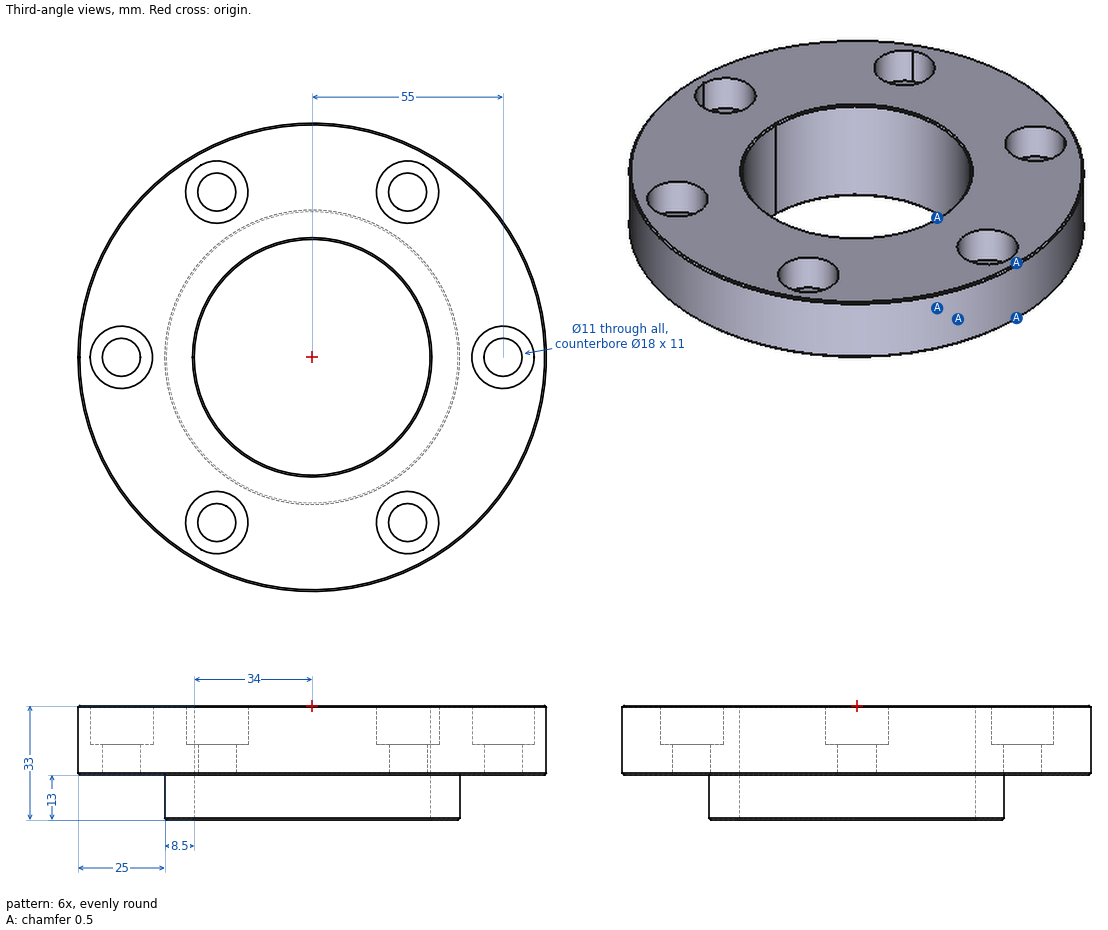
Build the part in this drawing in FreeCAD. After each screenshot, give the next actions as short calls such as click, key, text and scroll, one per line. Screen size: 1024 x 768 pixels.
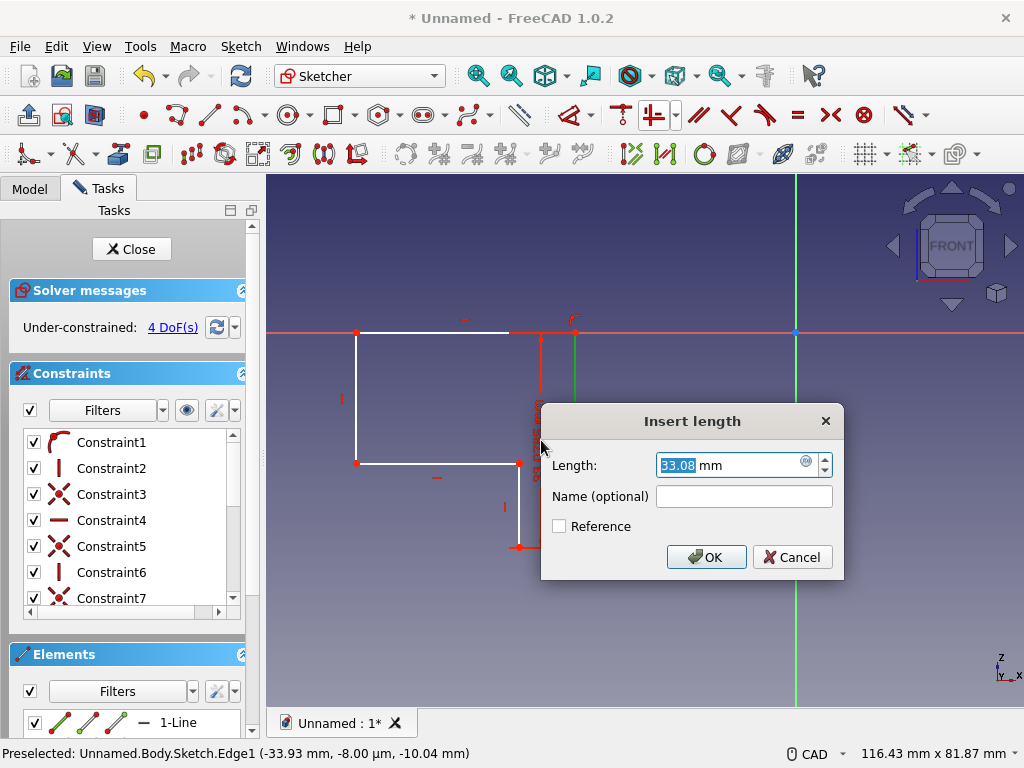
text(33)
key(Return)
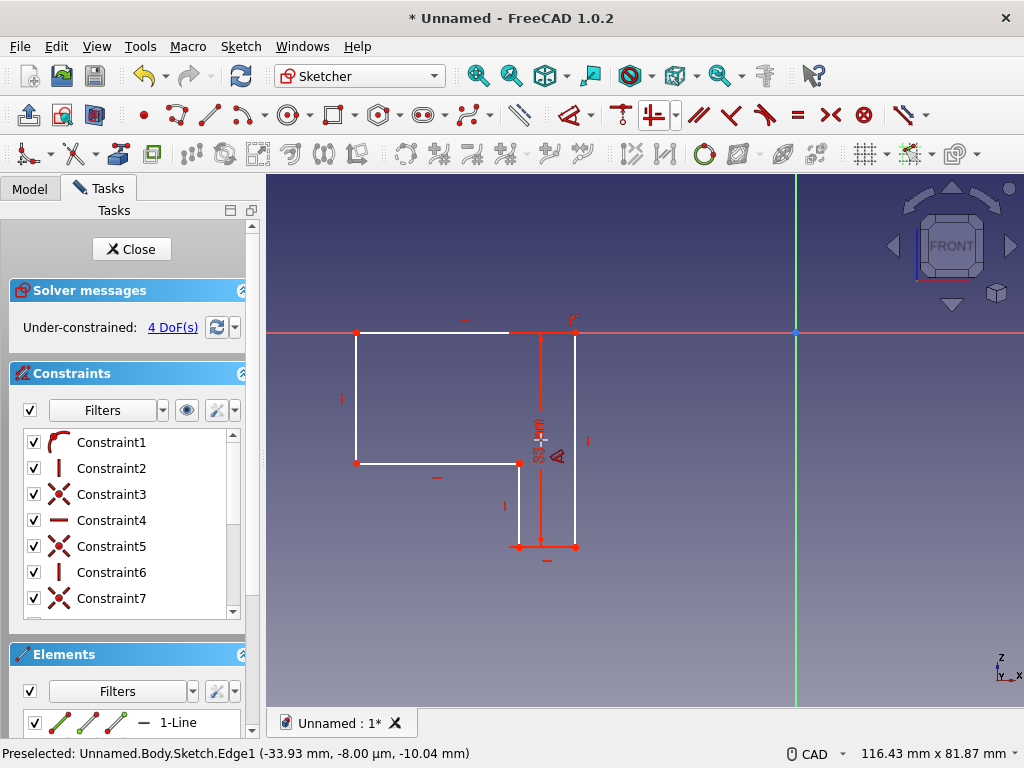
click(519, 522)
click(485, 506)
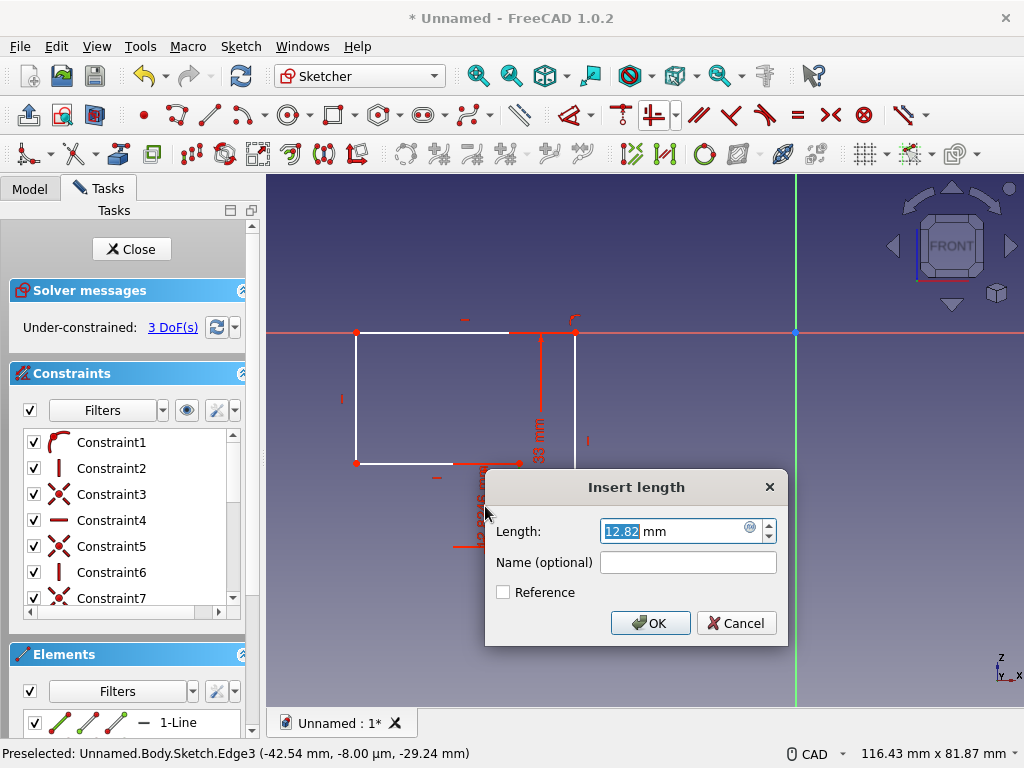
text(13)
key(Return)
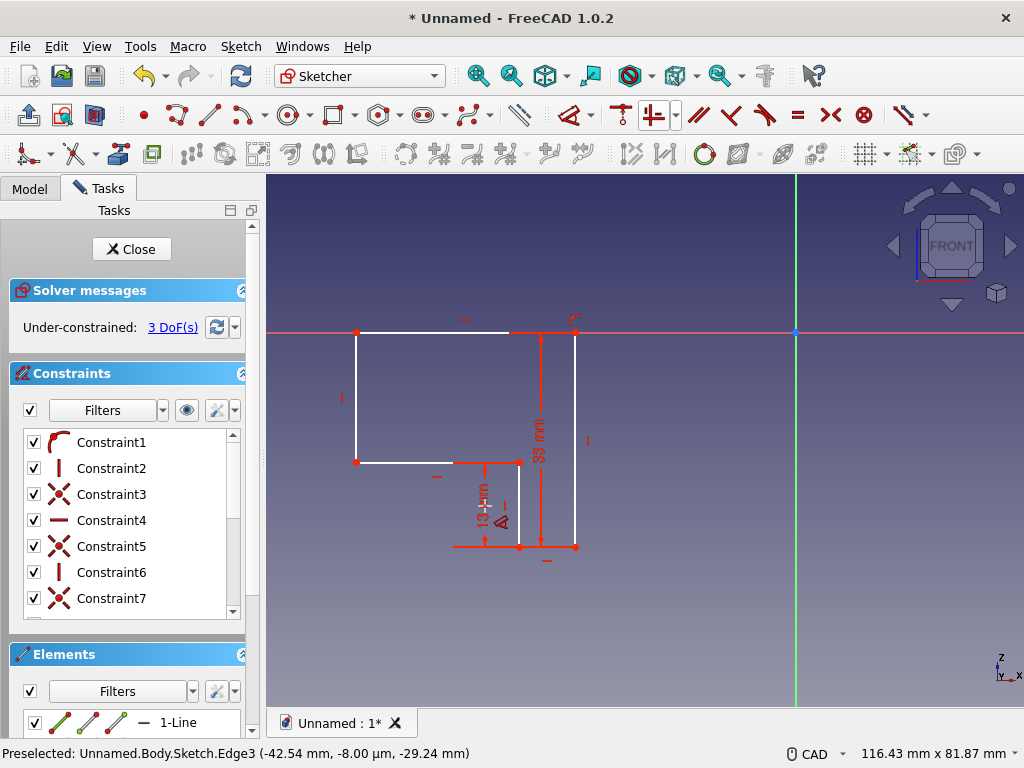
click(470, 463)
click(400, 497)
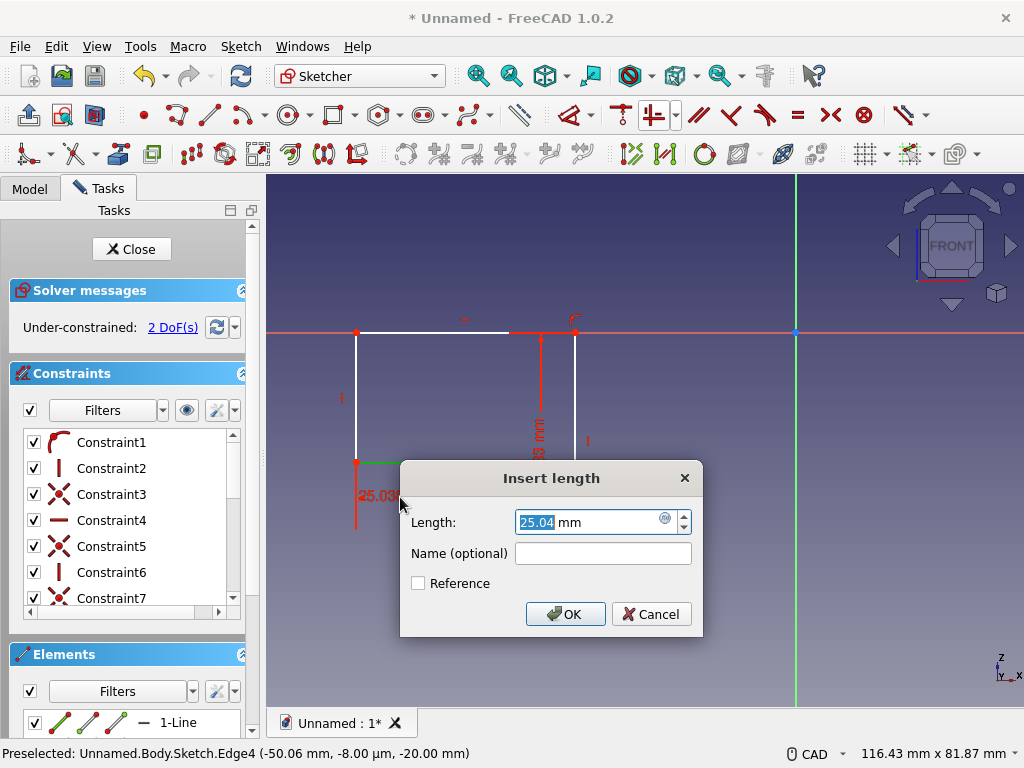
text(25)
key(Return)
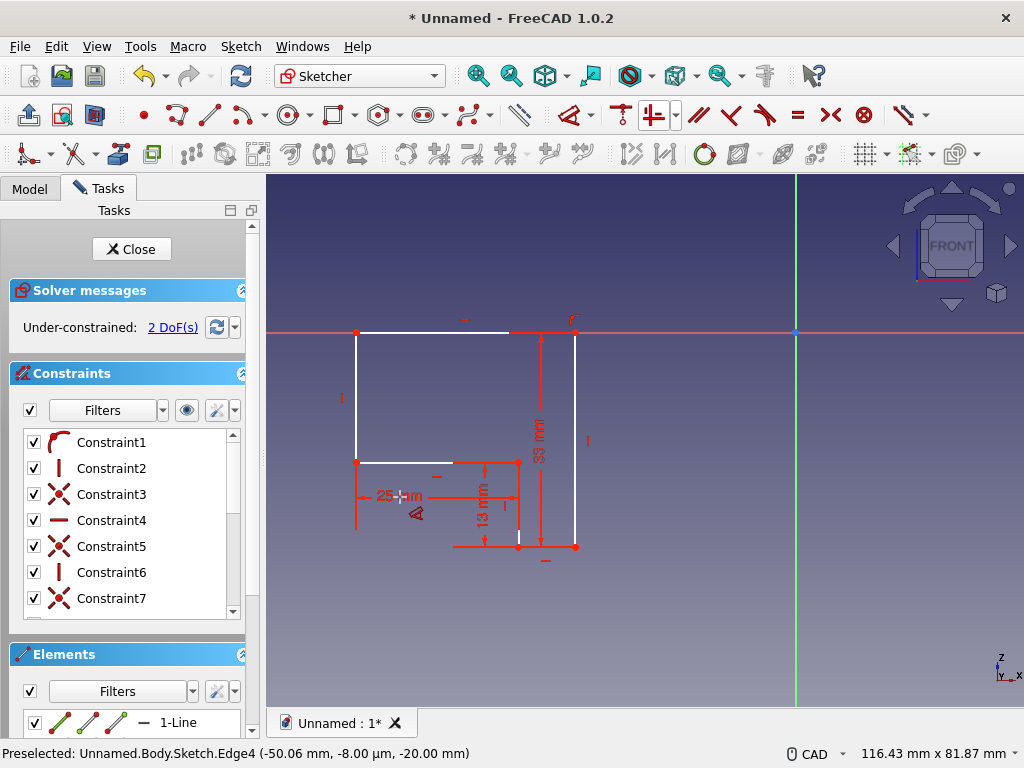
click(558, 547)
click(547, 581)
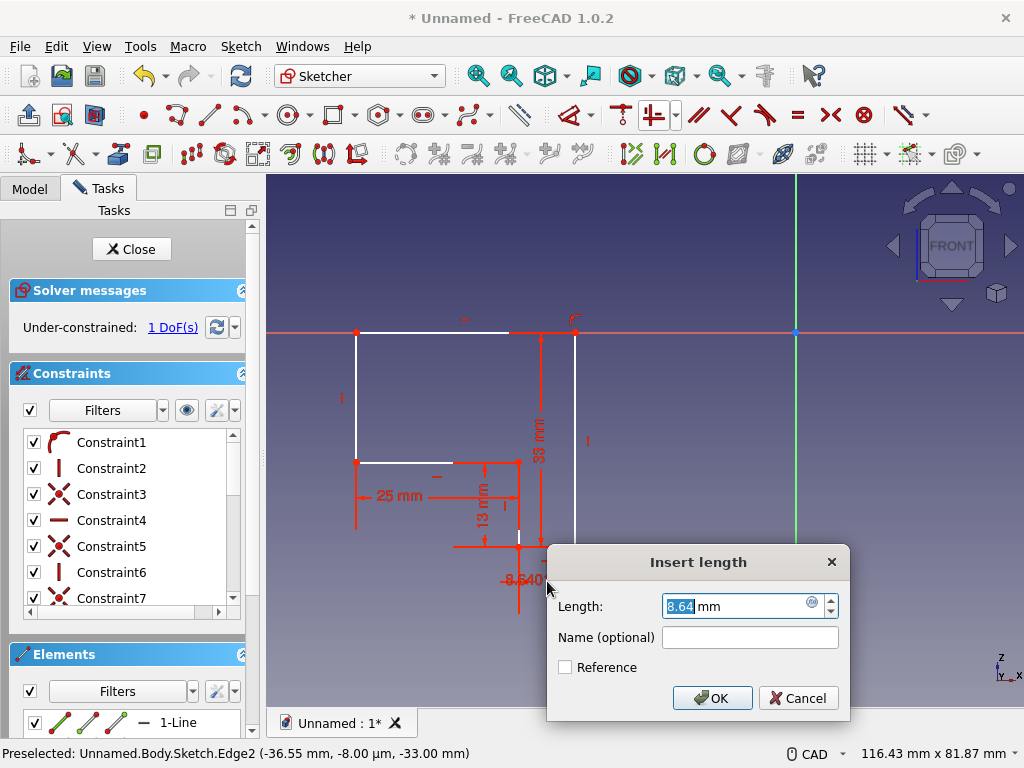
text(8.5)
key(Return)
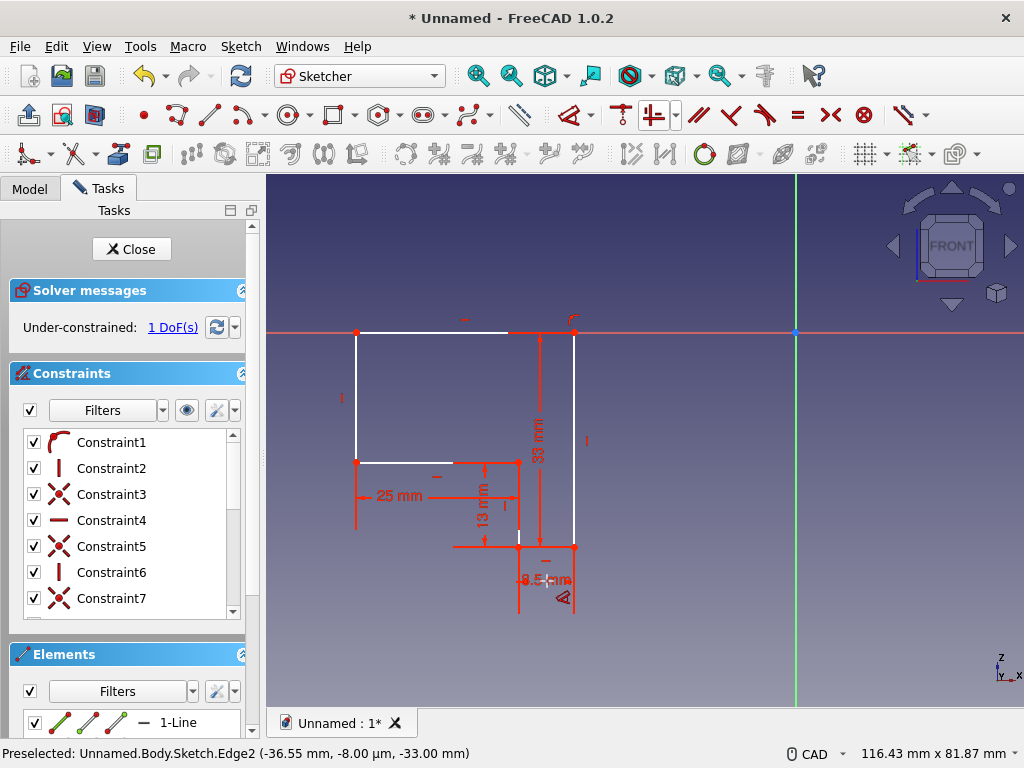
click(574, 333)
click(685, 299)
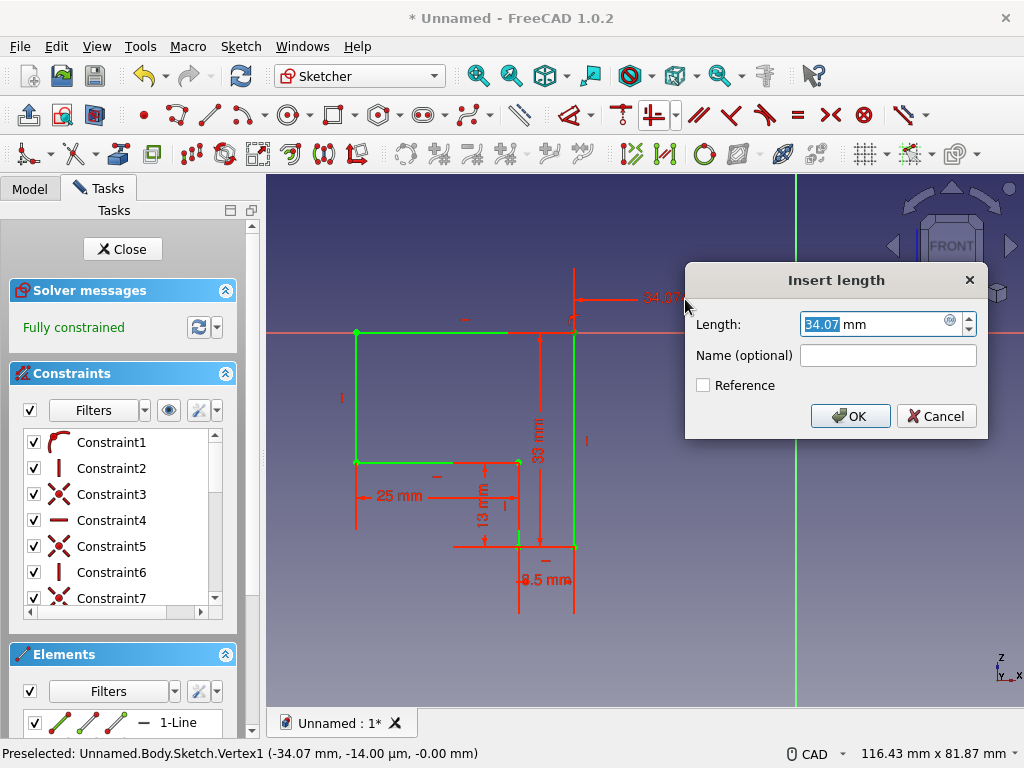
text(34)
key(Return)
key(Escape)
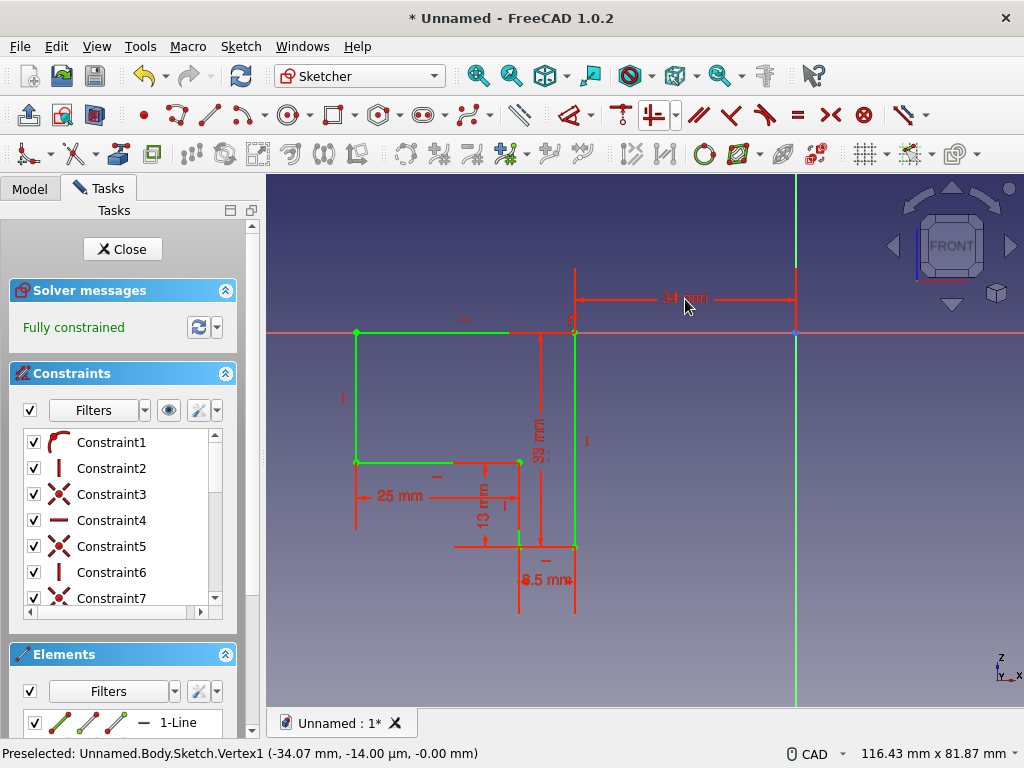
click(123, 249)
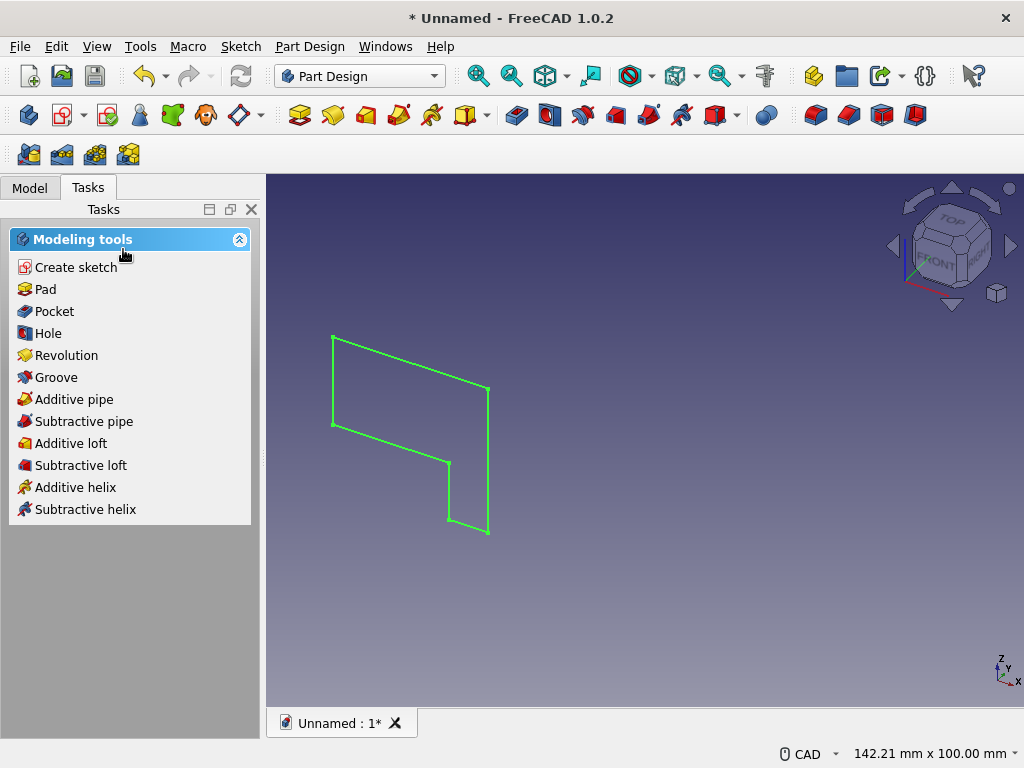
click(333, 116)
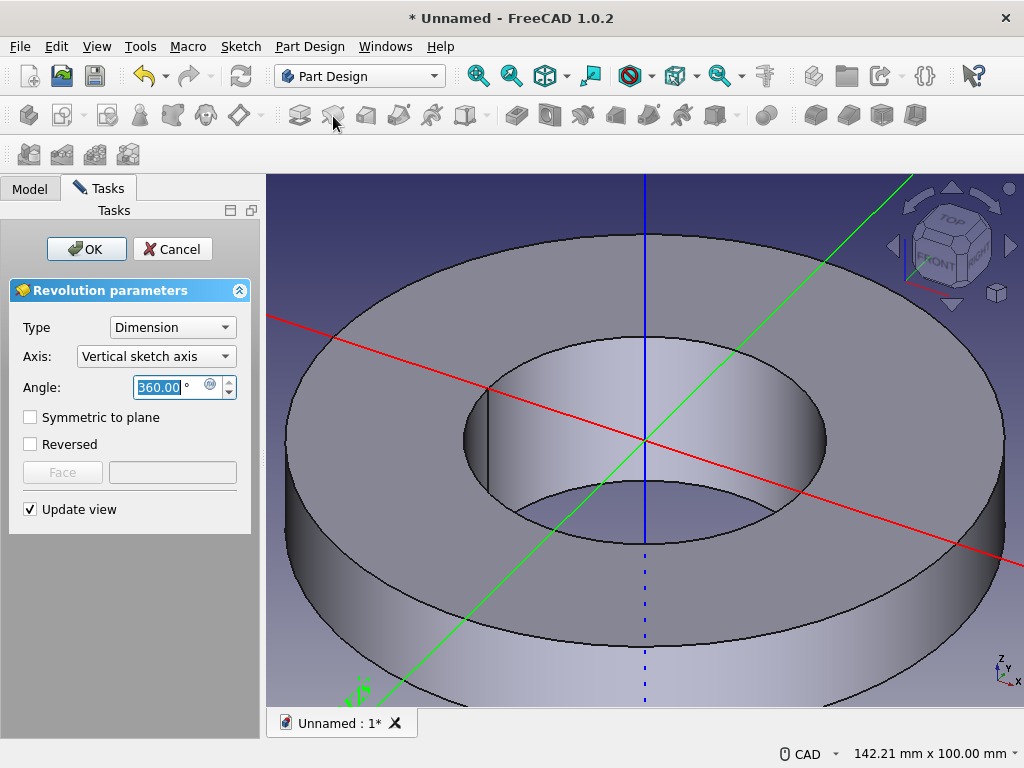
click(87, 249)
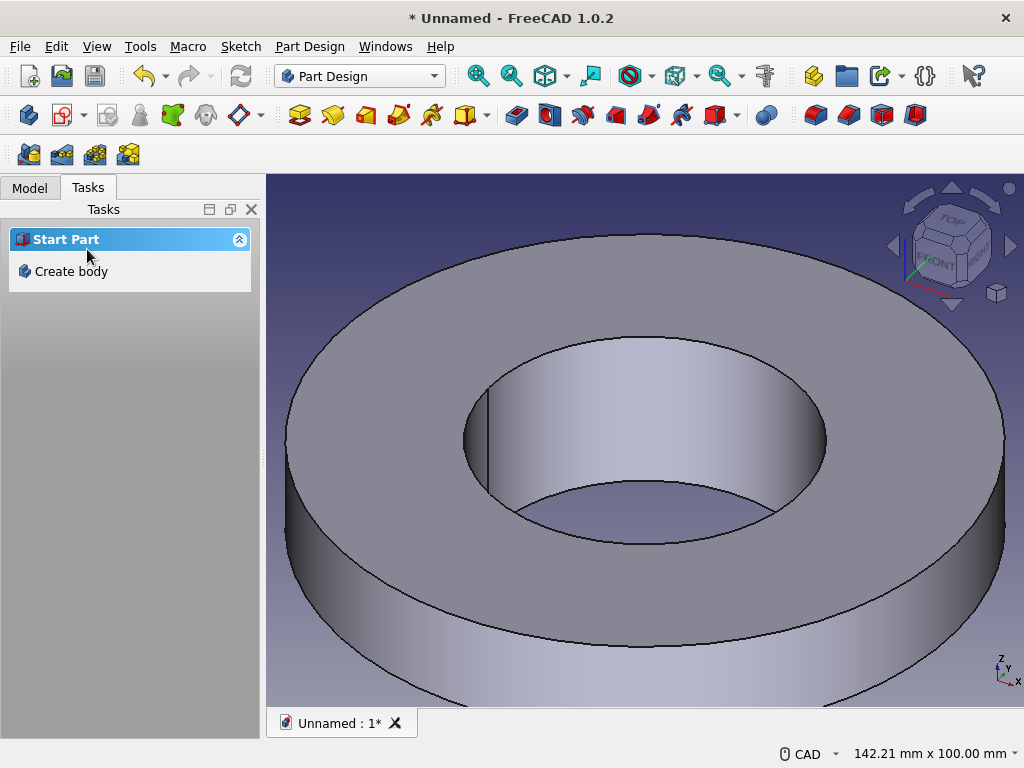
key(v)
key(f)